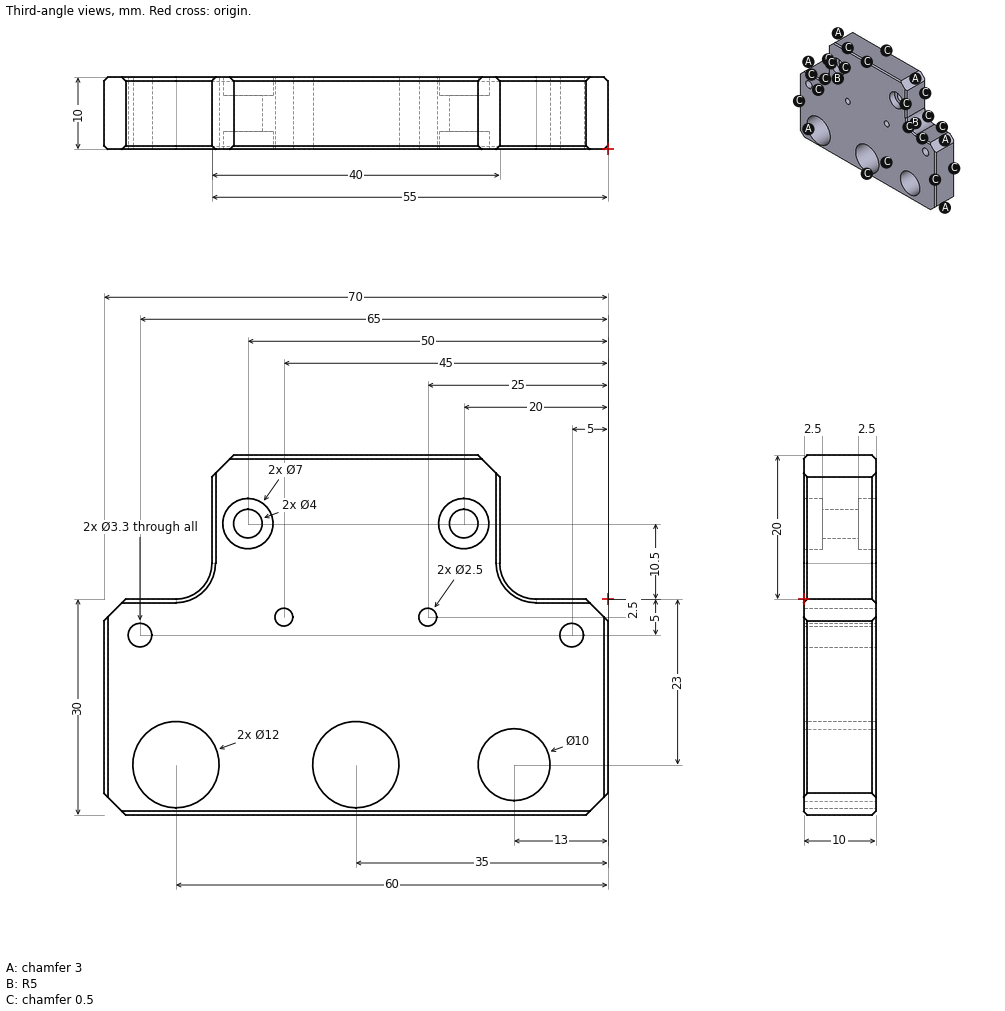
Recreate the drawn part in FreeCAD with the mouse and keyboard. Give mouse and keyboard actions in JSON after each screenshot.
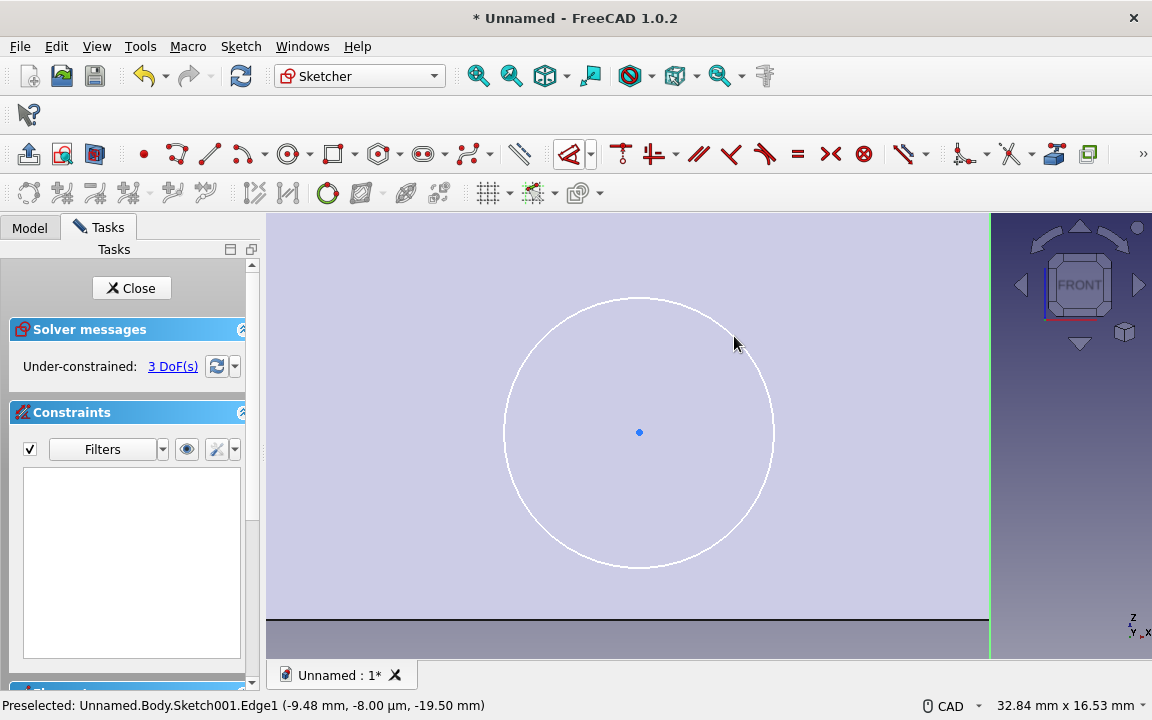
{"action": "left_click", "coordinate": [734, 337]}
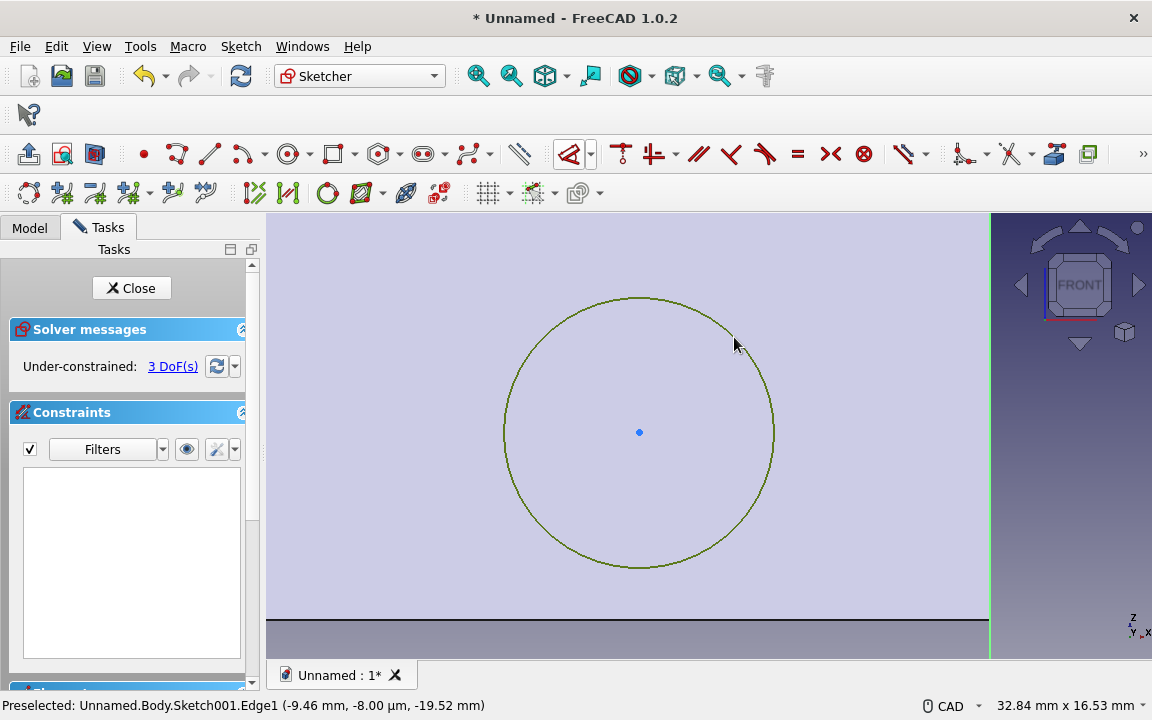
{"action": "left_click", "coordinate": [590, 154]}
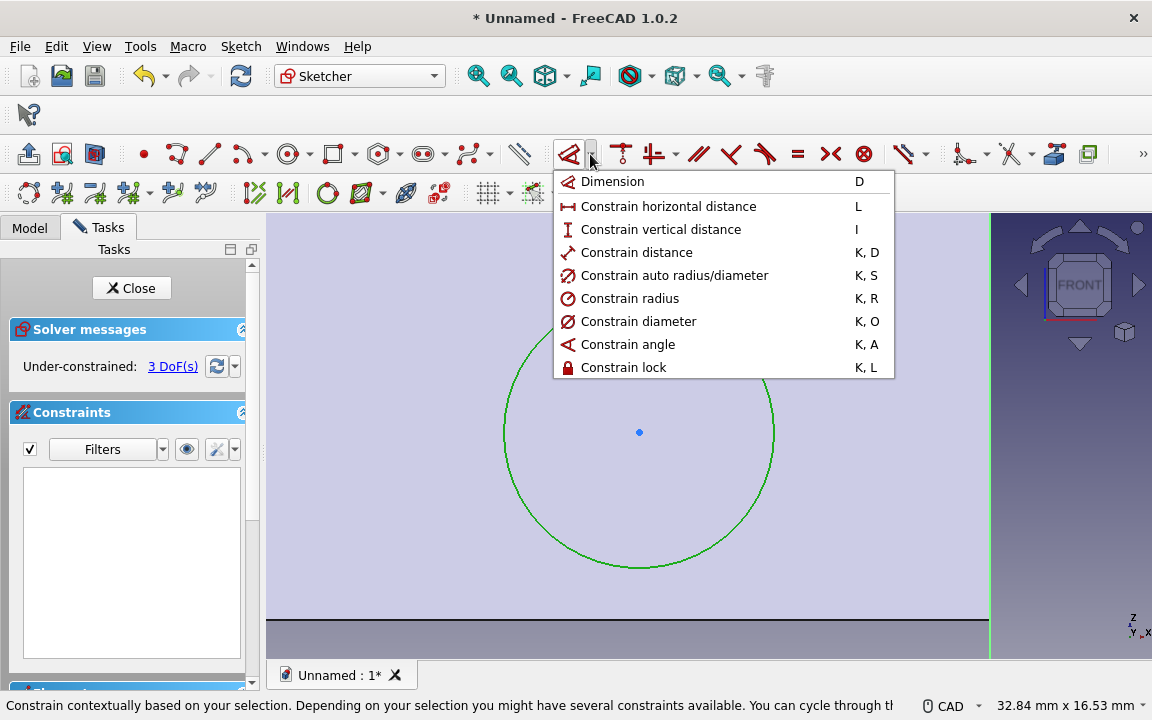
{"action": "left_click", "coordinate": [724, 322]}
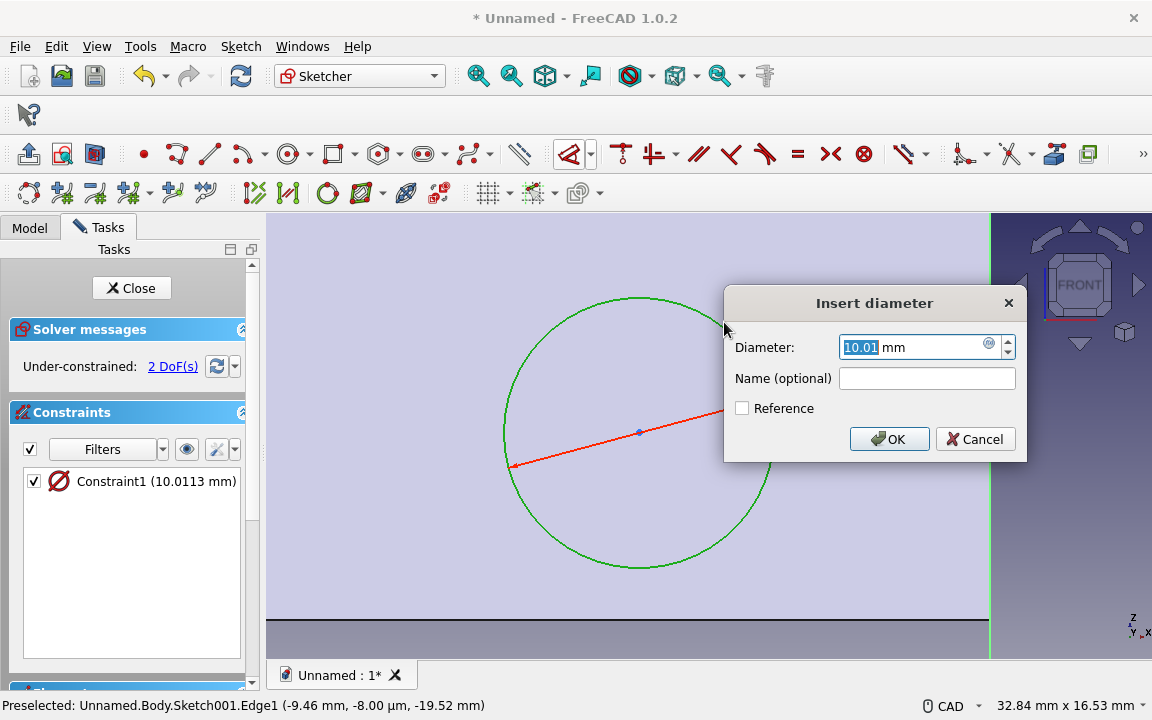
{"action": "type", "text": "10"}
{"action": "key", "text": "Return"}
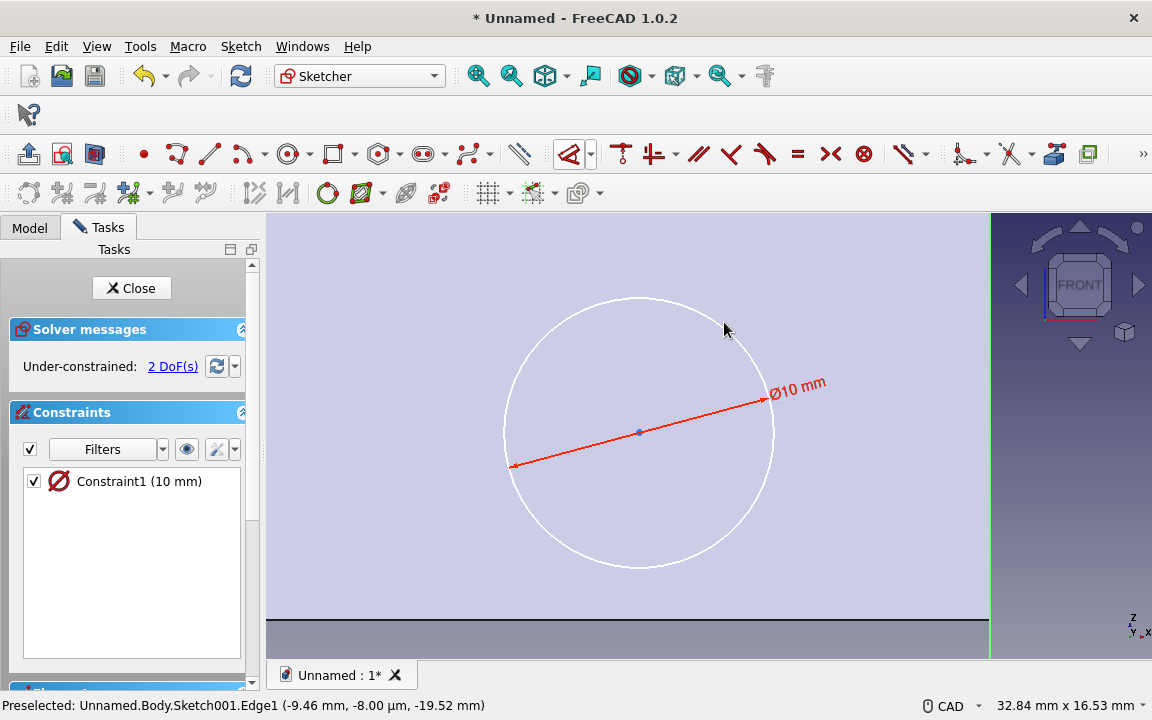
{"action": "left_click", "coordinate": [639, 433]}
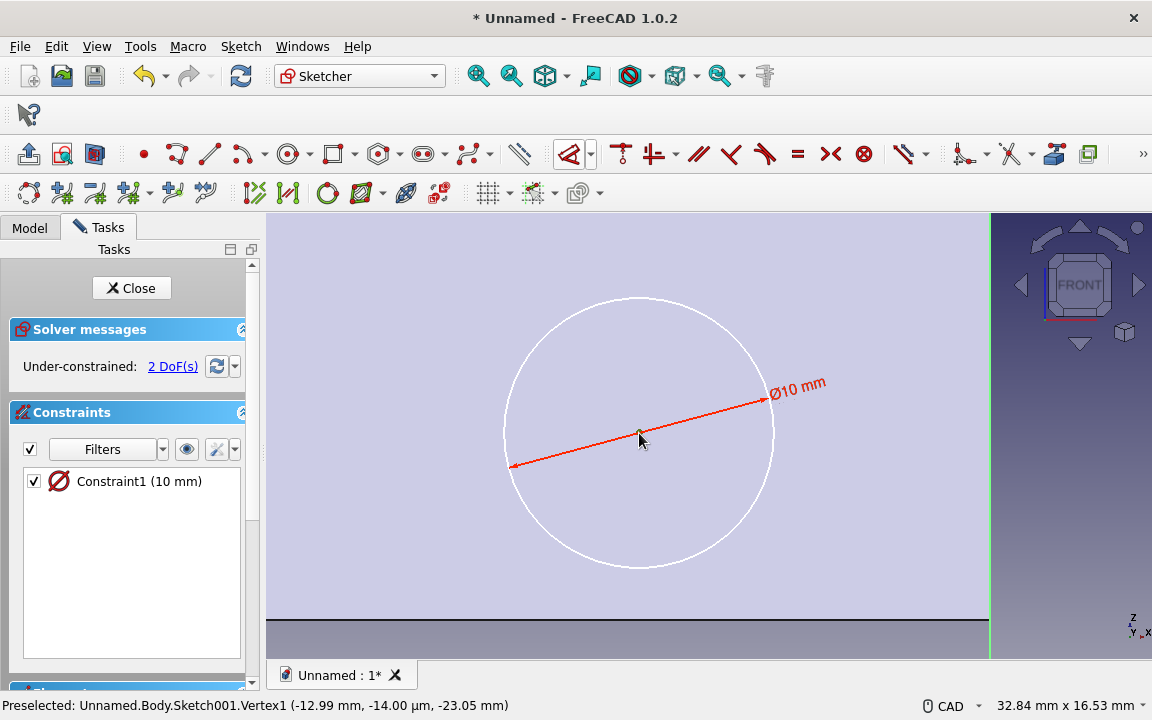
{"action": "left_click", "coordinate": [590, 154]}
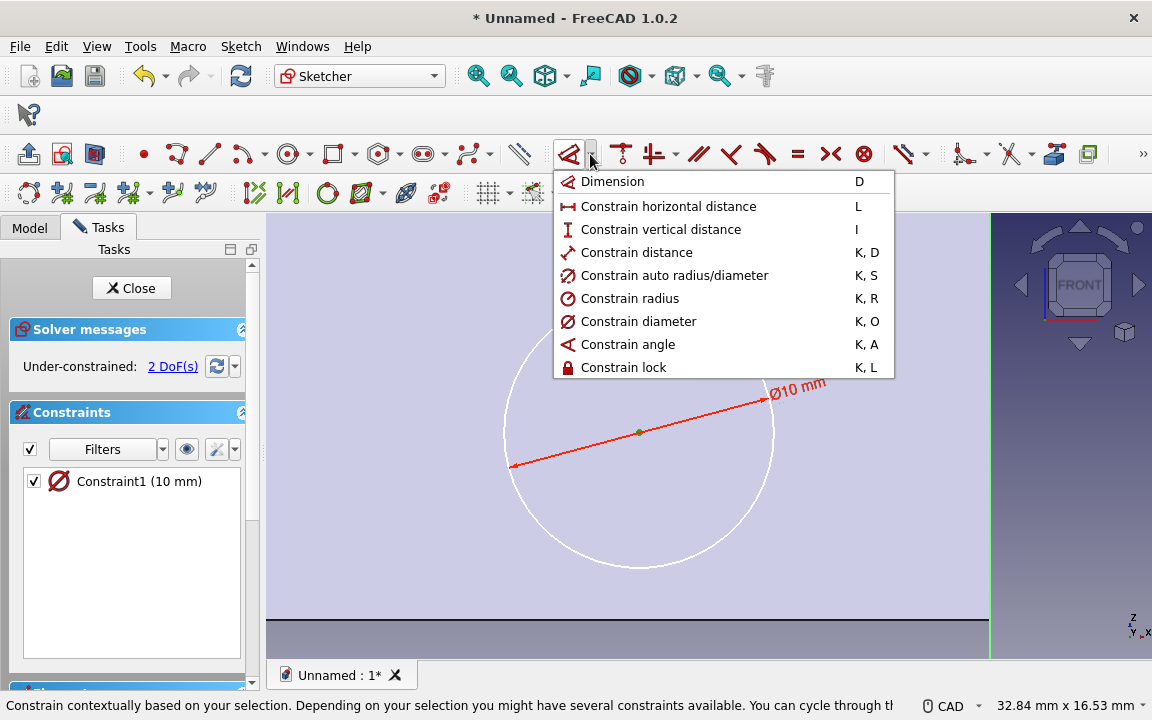
{"action": "left_click", "coordinate": [724, 206]}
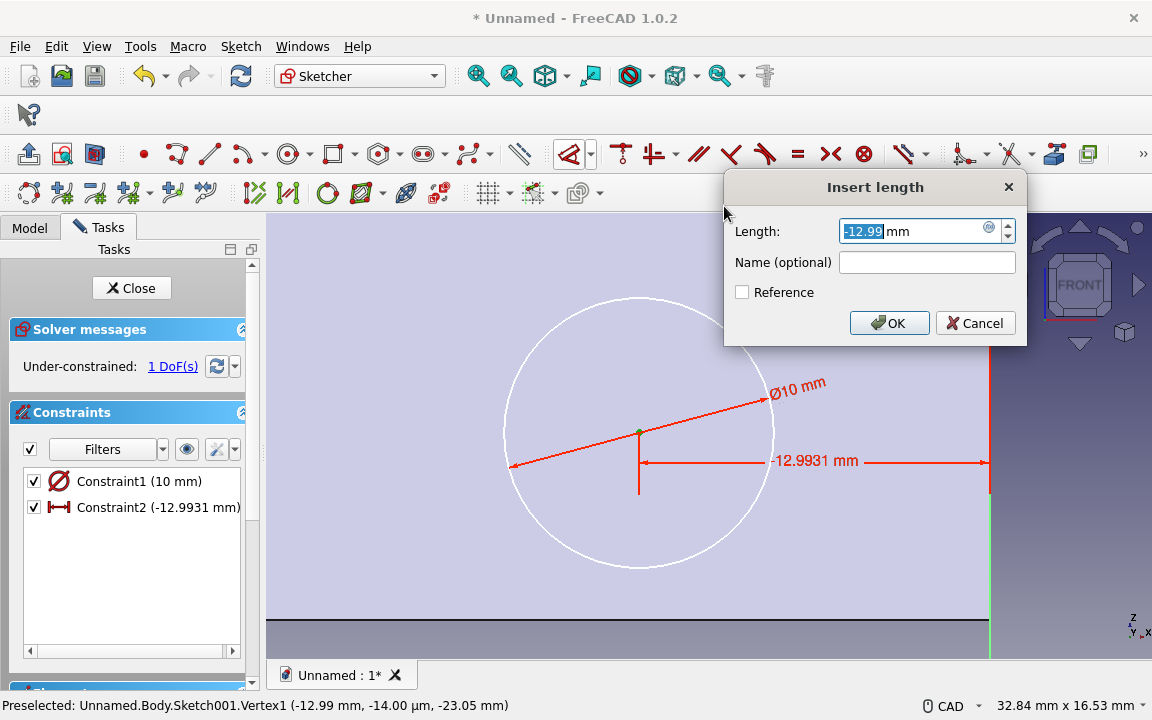
{"action": "type", "text": "-13"}
{"action": "key", "text": "Return"}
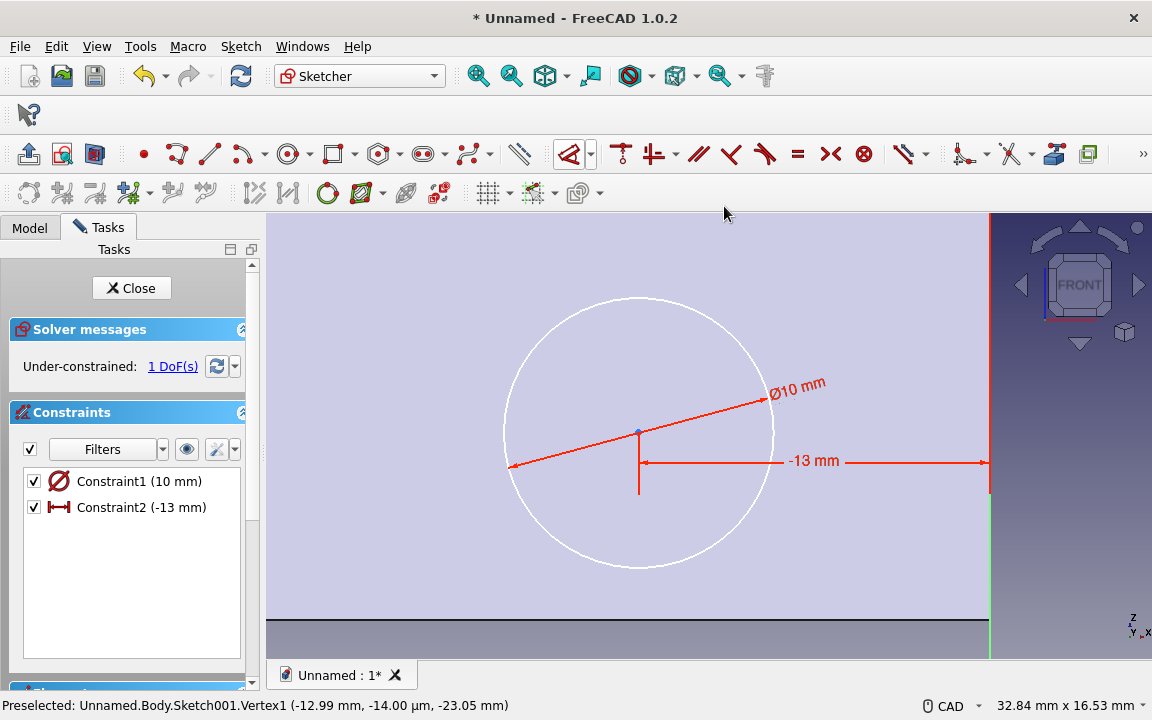
{"action": "left_click", "coordinate": [639, 433]}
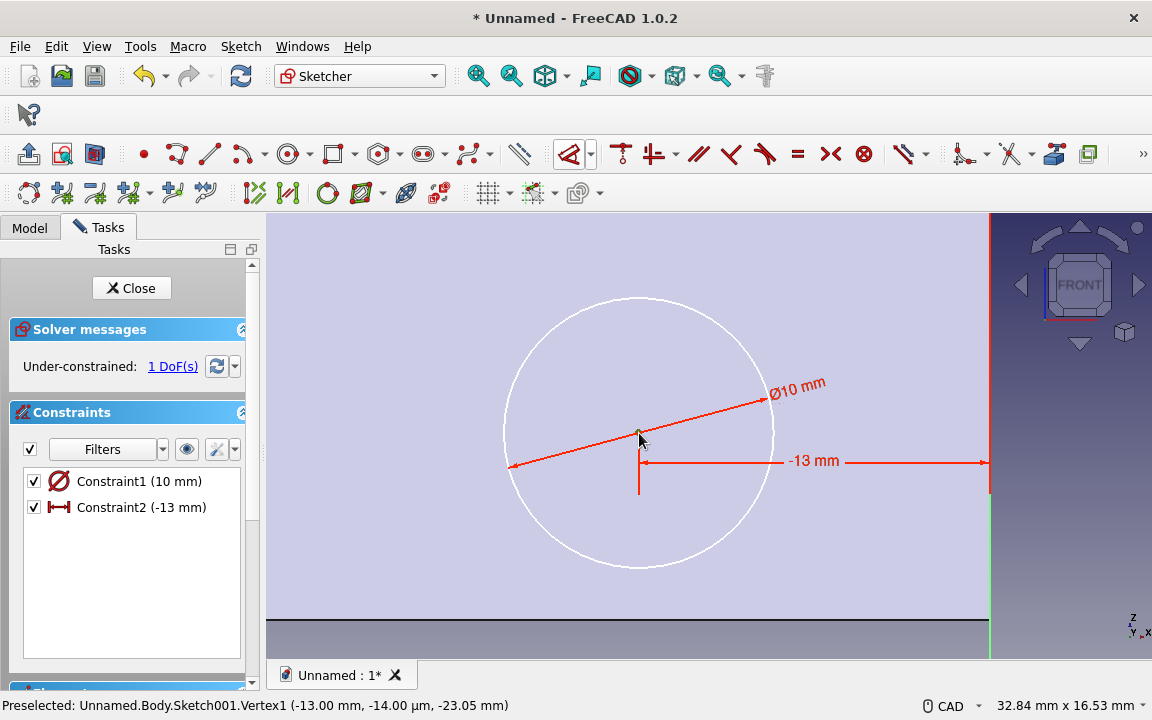
{"action": "key", "text": "i"}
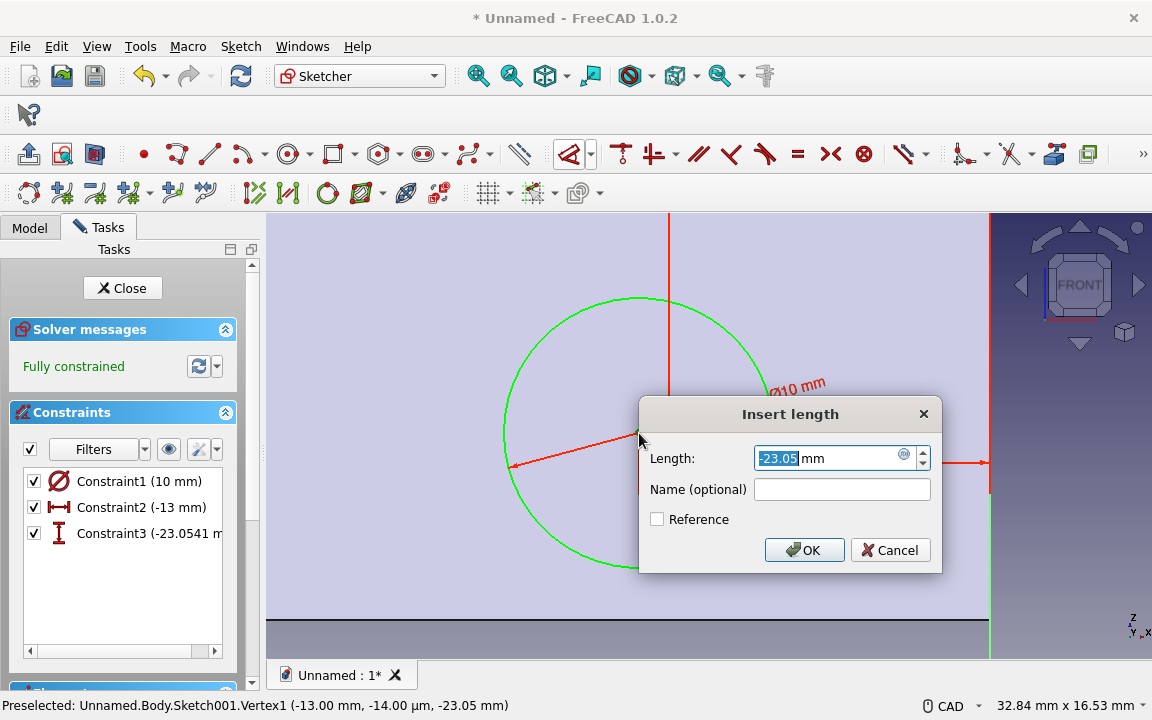
{"action": "type", "text": "-23"}
{"action": "key", "text": "Return"}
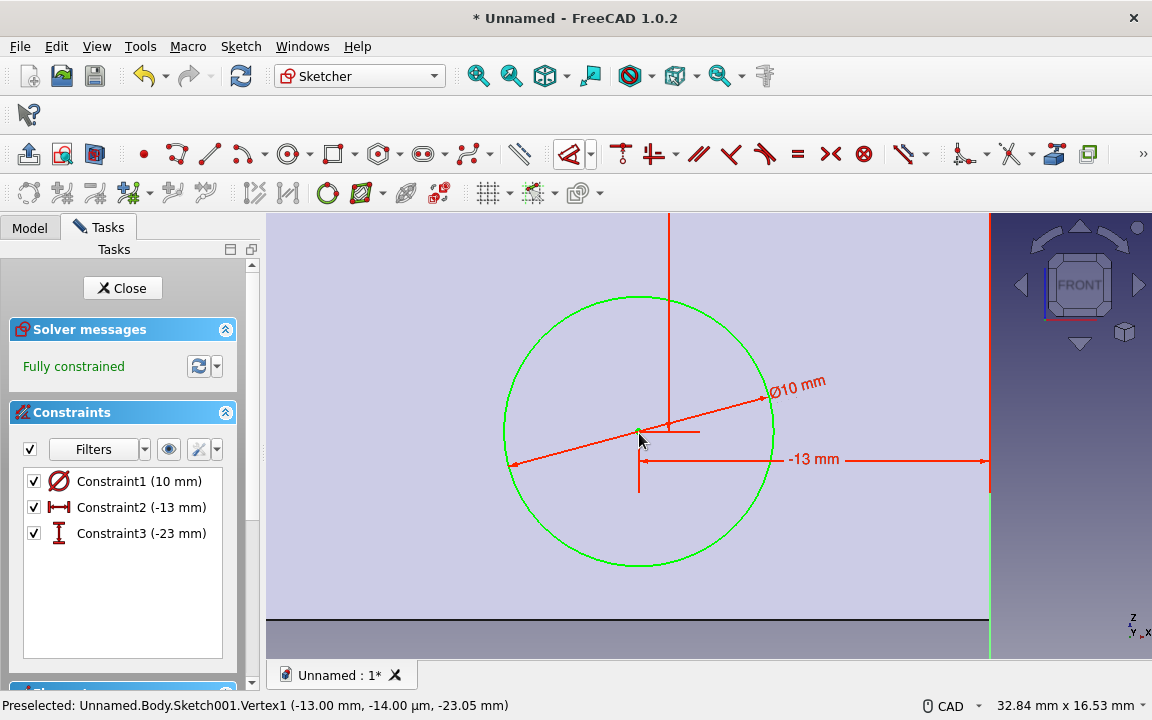
{"action": "left_click", "coordinate": [123, 288]}